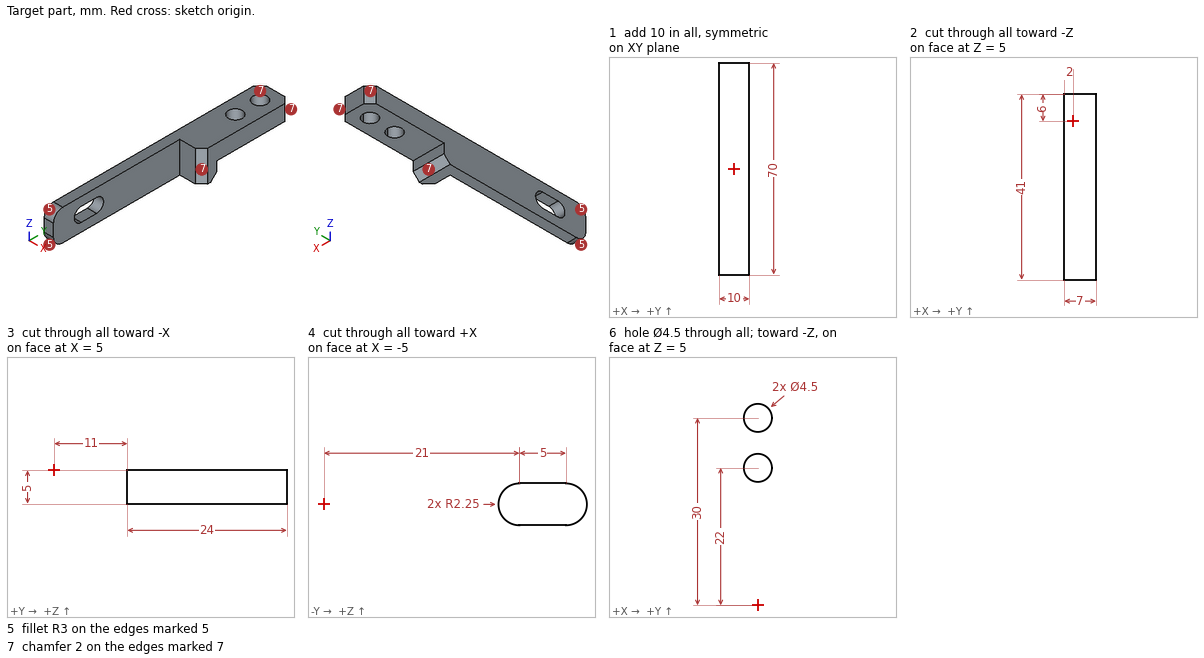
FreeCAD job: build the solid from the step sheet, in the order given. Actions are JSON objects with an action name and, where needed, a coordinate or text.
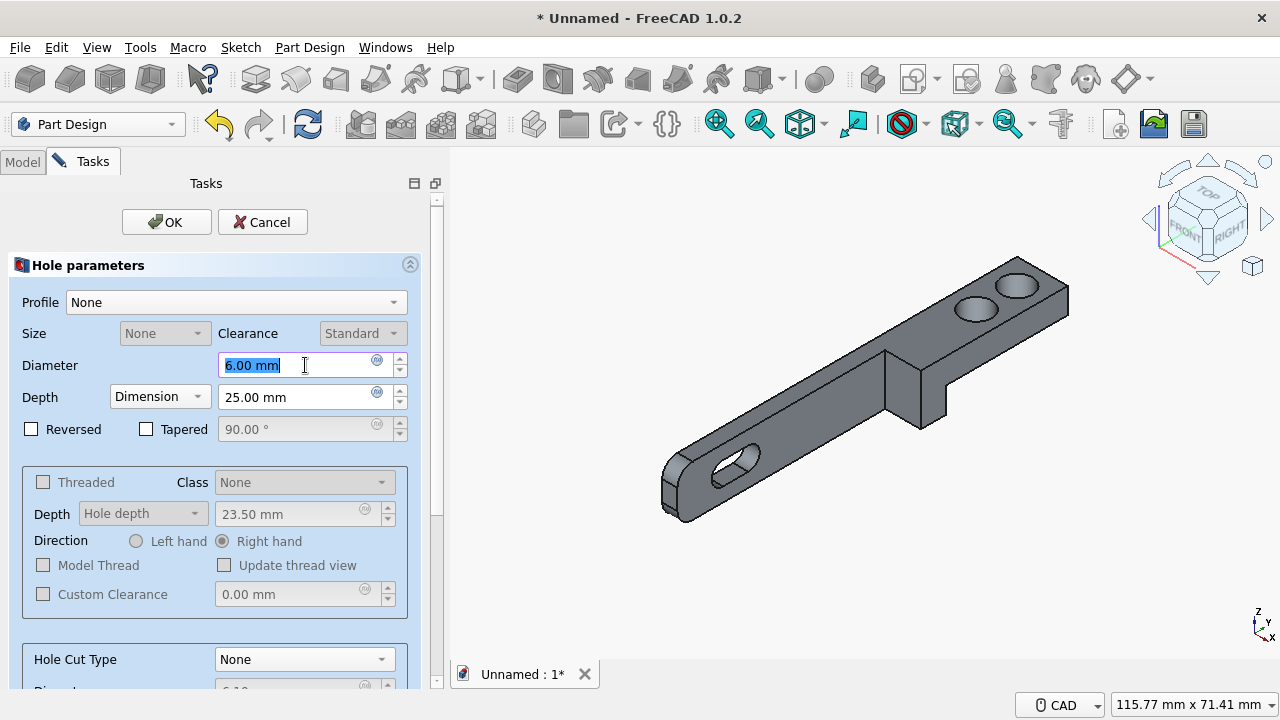
{"action": "type", "text": "4.5"}
{"action": "key", "text": "Tab"}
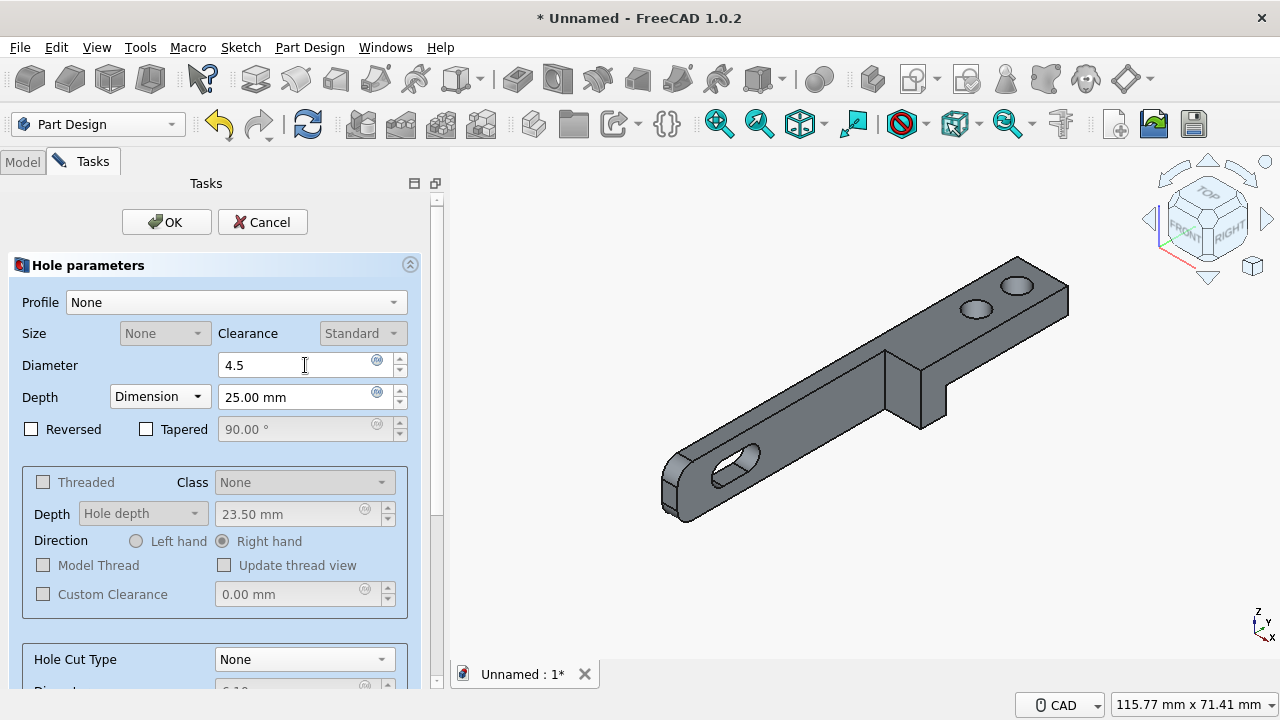
{"action": "left_click", "coordinate": [161, 396]}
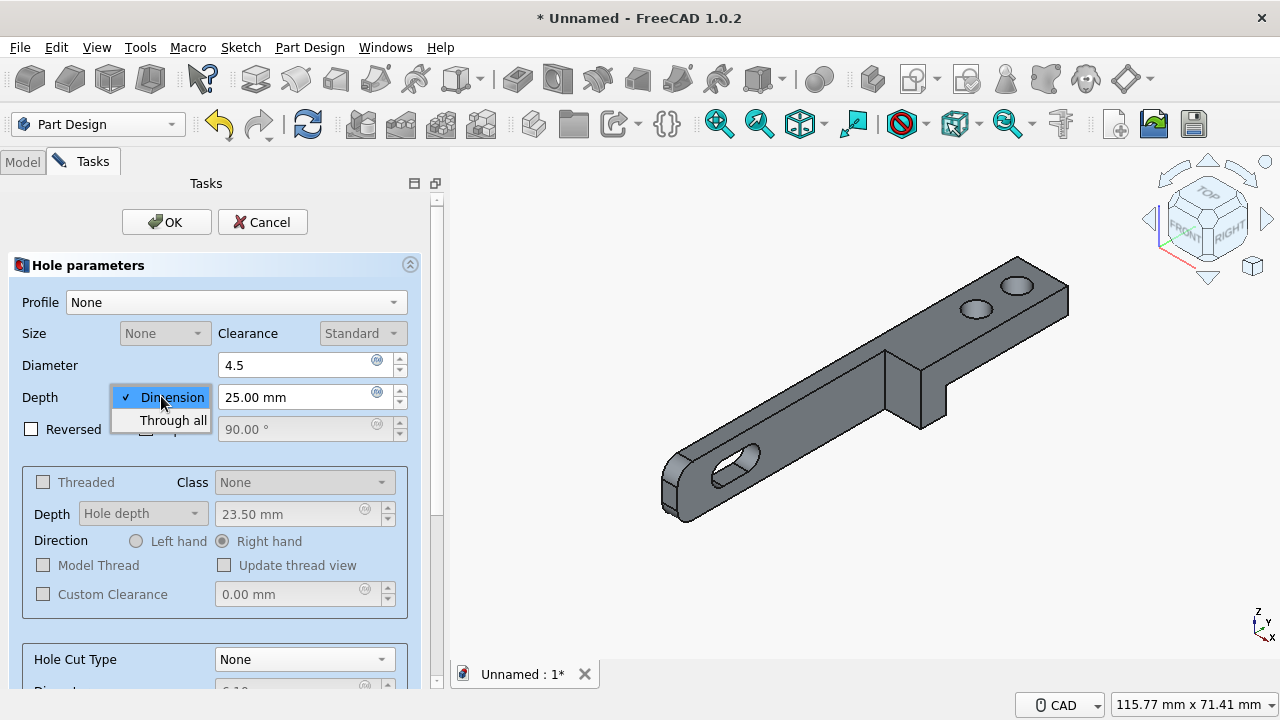
{"action": "left_click", "coordinate": [160, 420]}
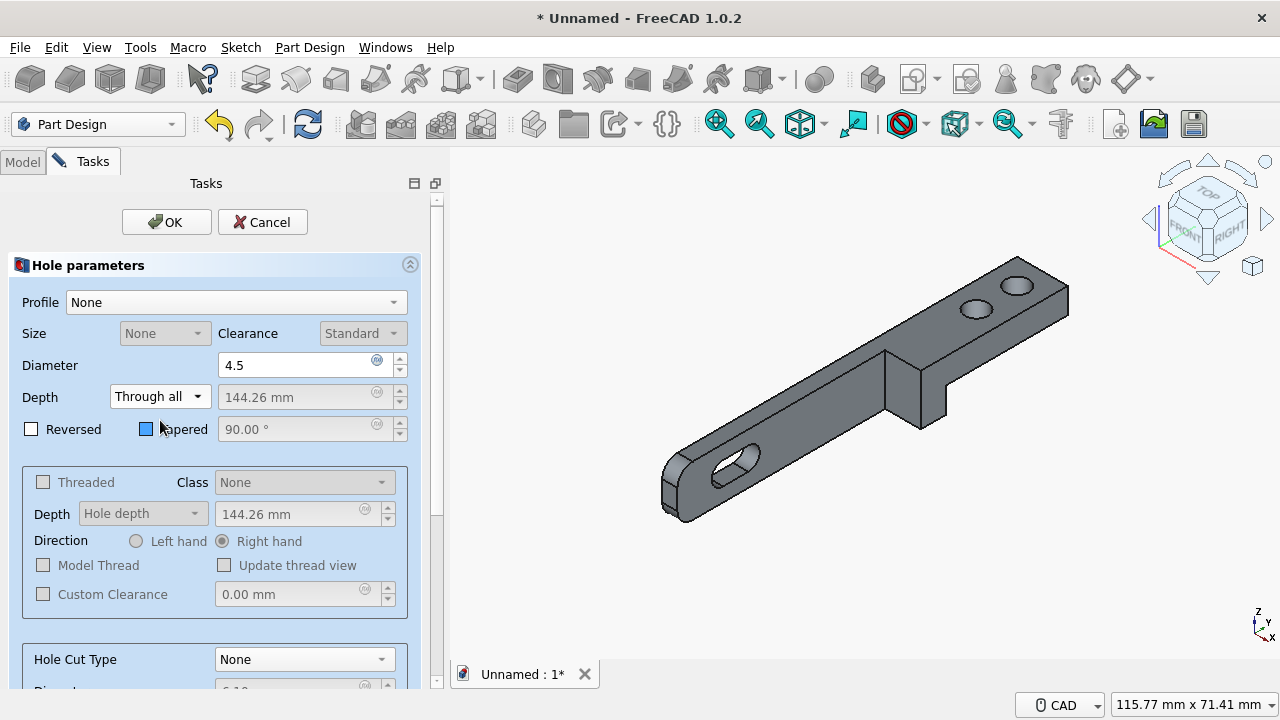
{"action": "left_click", "coordinate": [167, 222]}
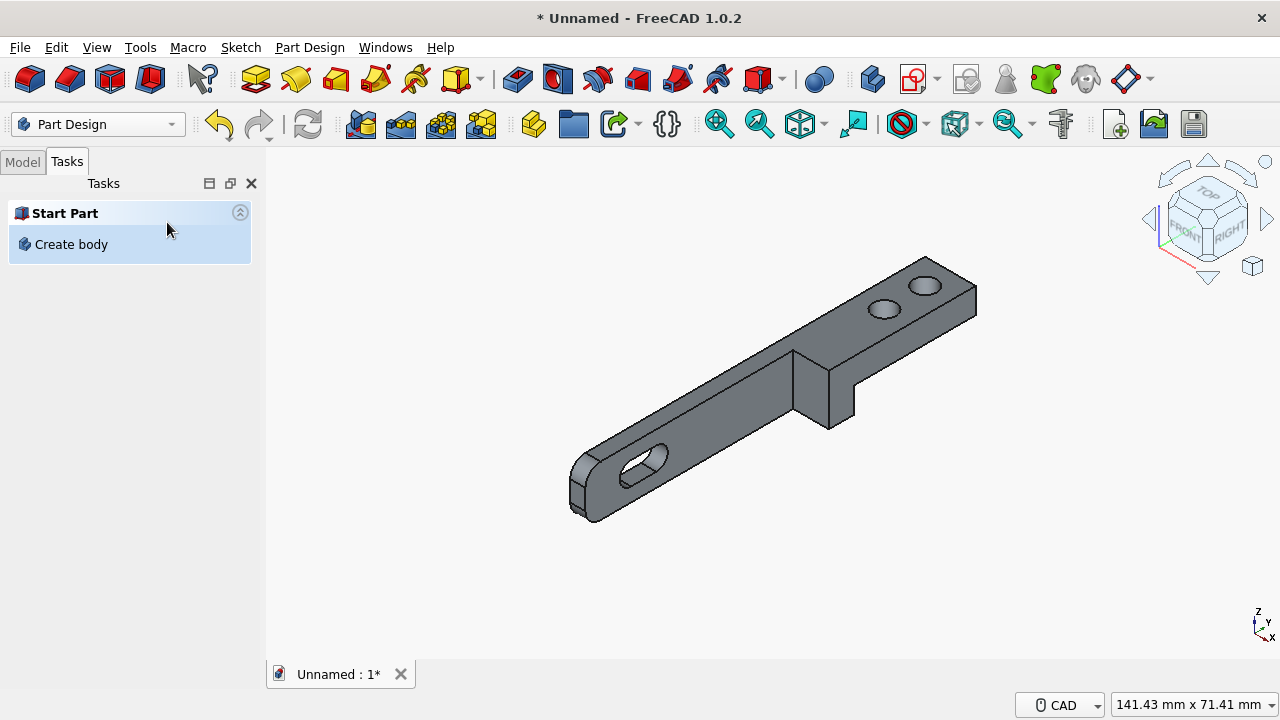
{"action": "left_click", "coordinate": [829, 399]}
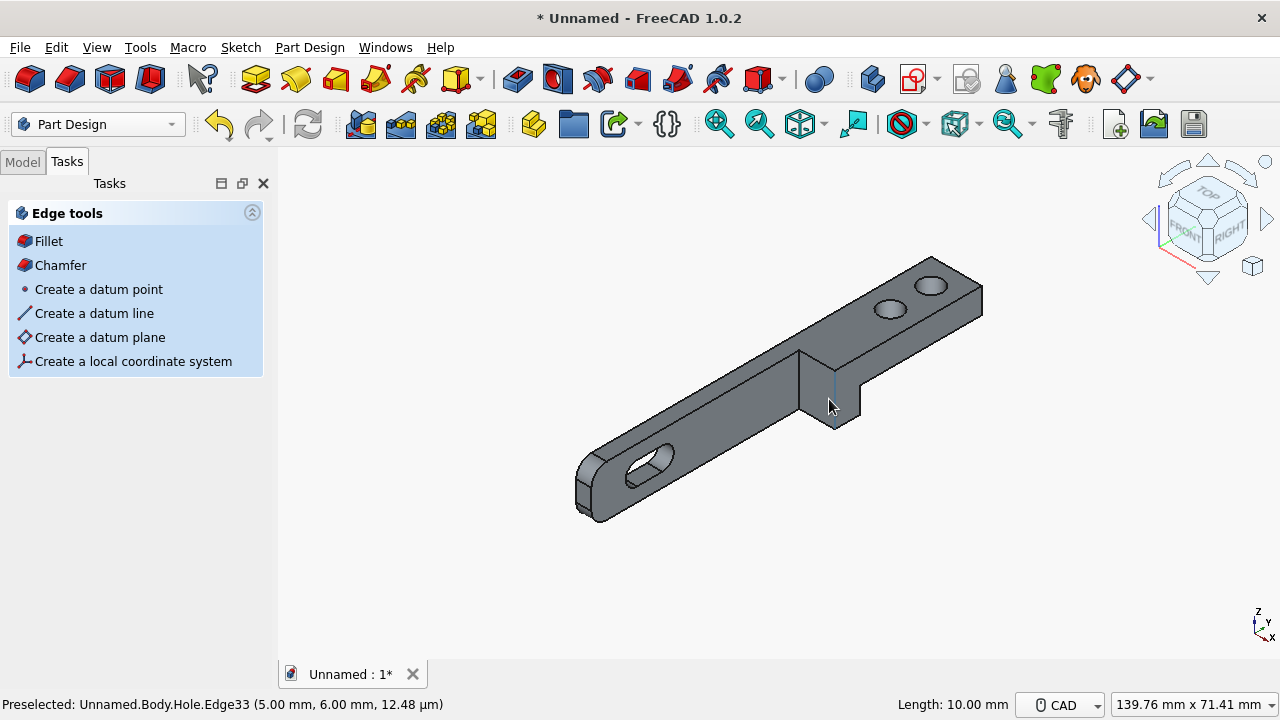
{"action": "key", "text": "2"}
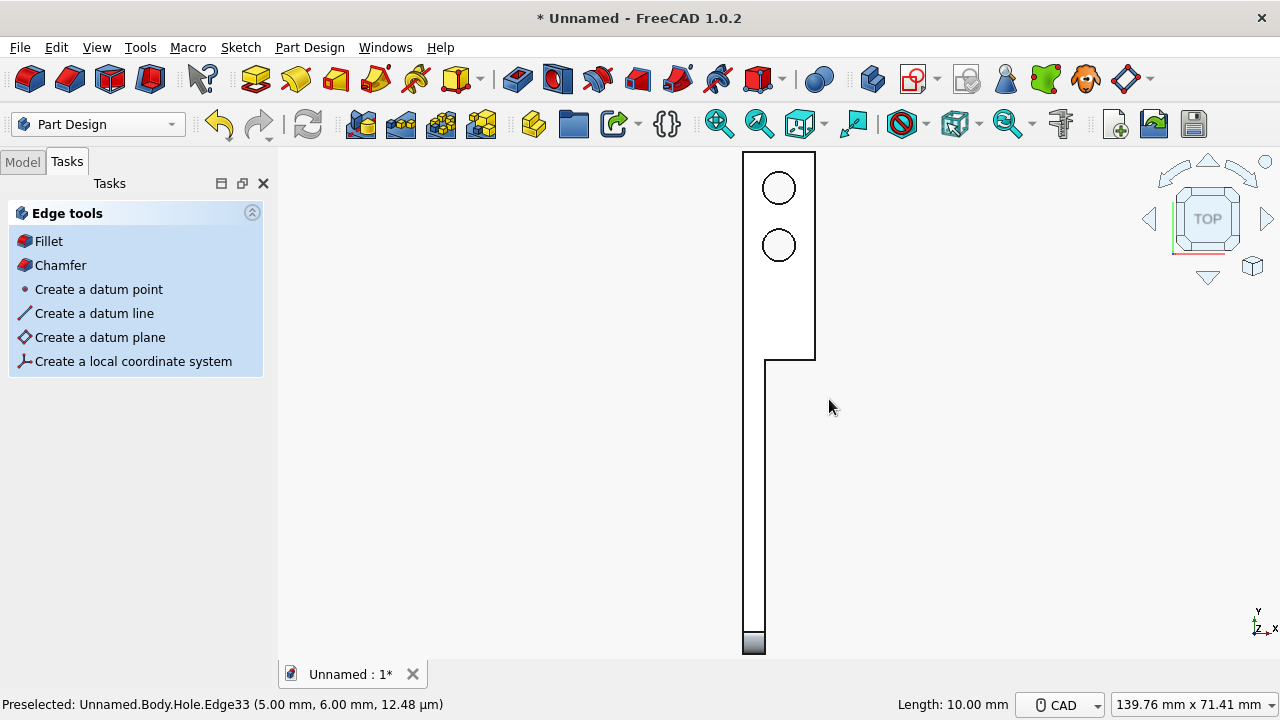
{"action": "key", "text": "0"}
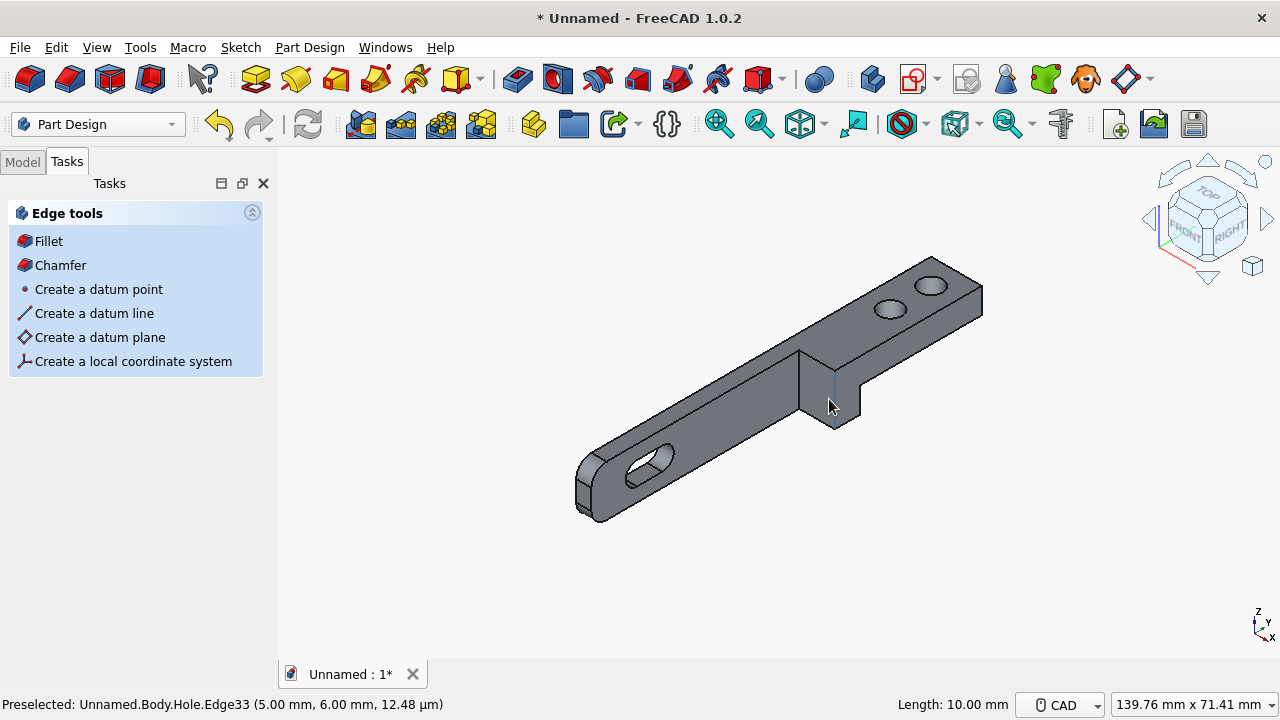
{"action": "key", "text": "1"}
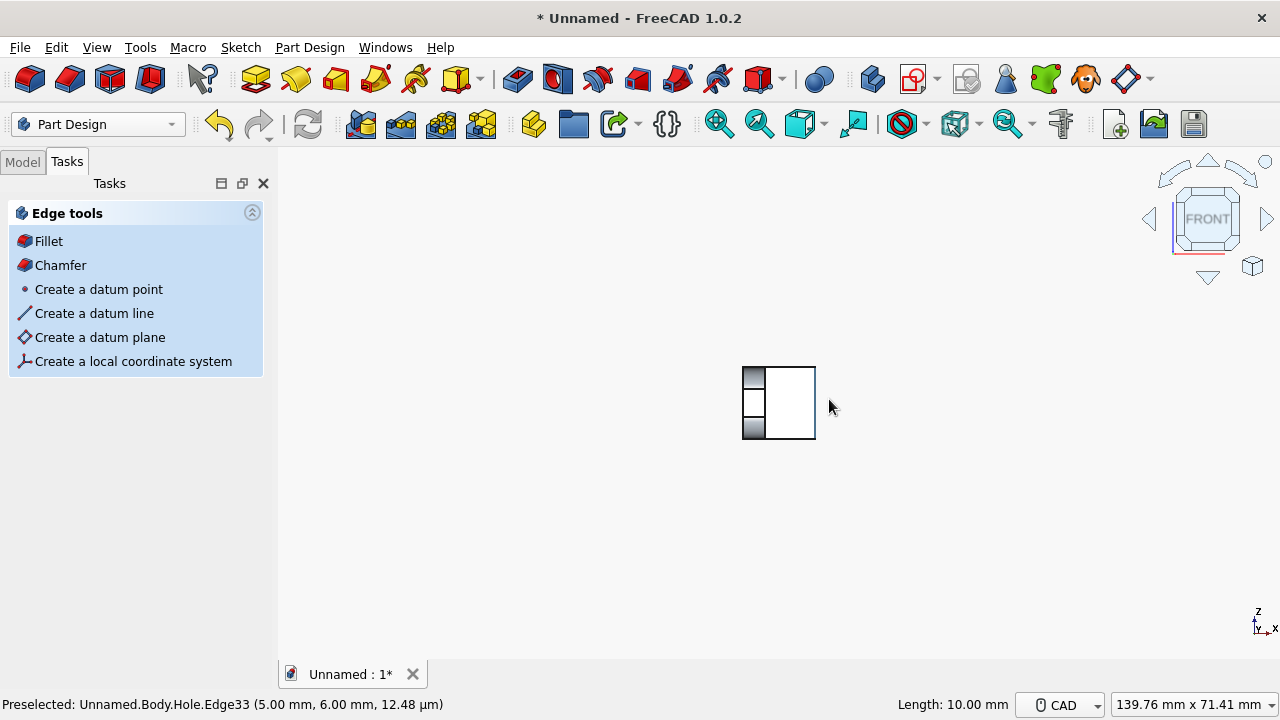
{"action": "key", "text": "v f"}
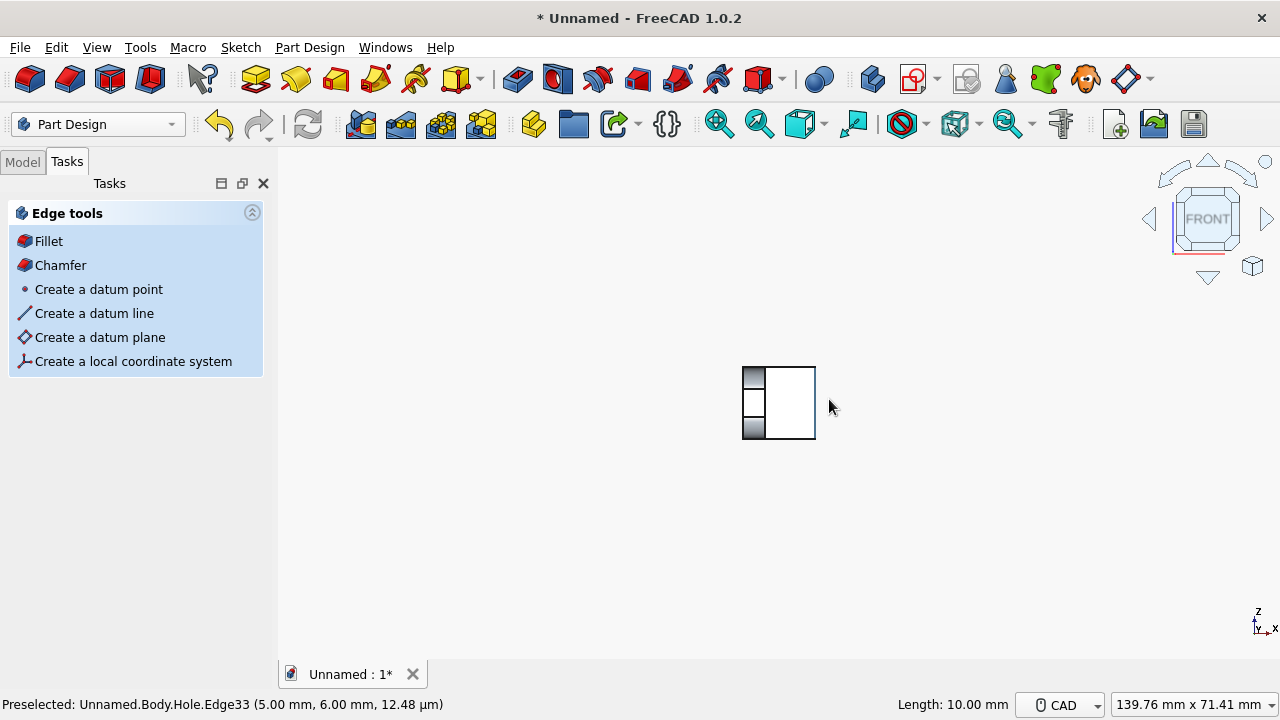
{"action": "key", "text": "3"}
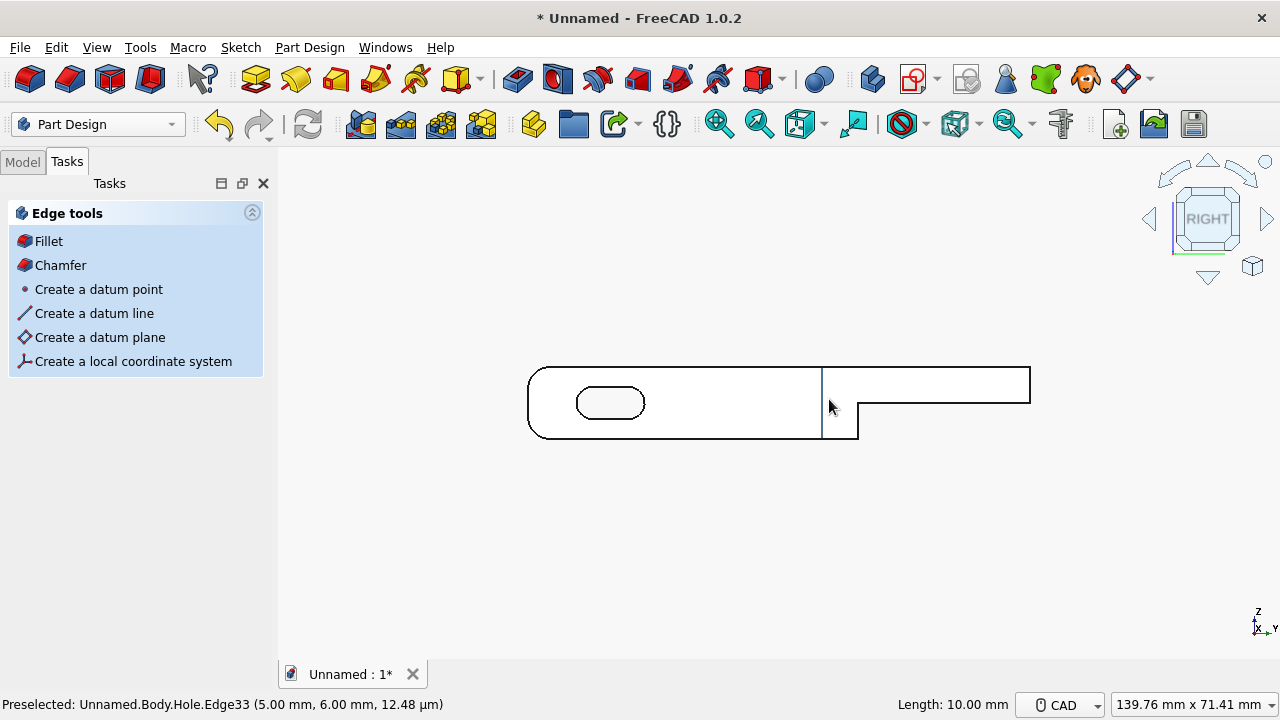
{"action": "left_click", "coordinate": [1030, 384], "text": "ctrl"}